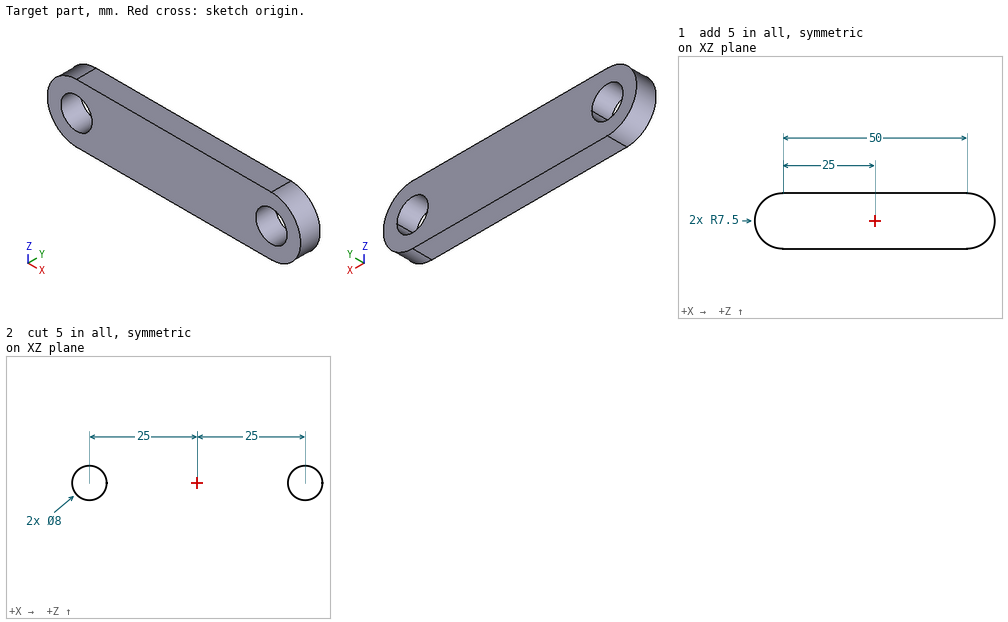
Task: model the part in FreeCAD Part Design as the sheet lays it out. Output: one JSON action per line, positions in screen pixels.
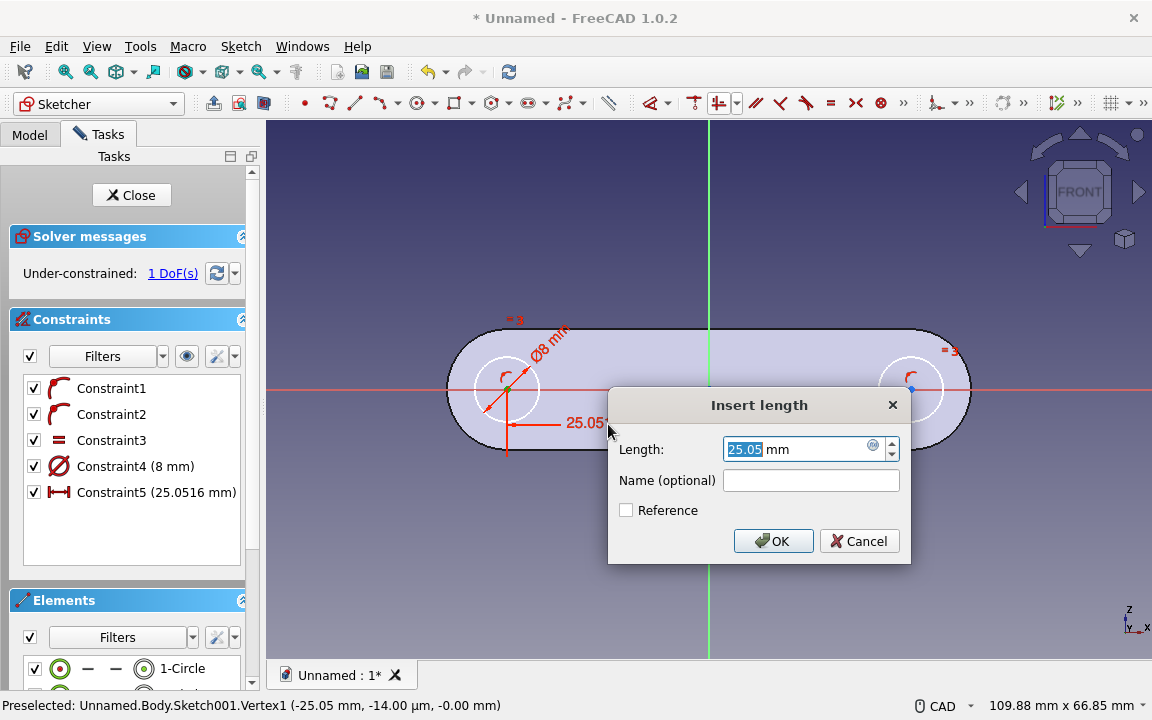
{"action": "type", "text": "25"}
{"action": "key", "text": "Return"}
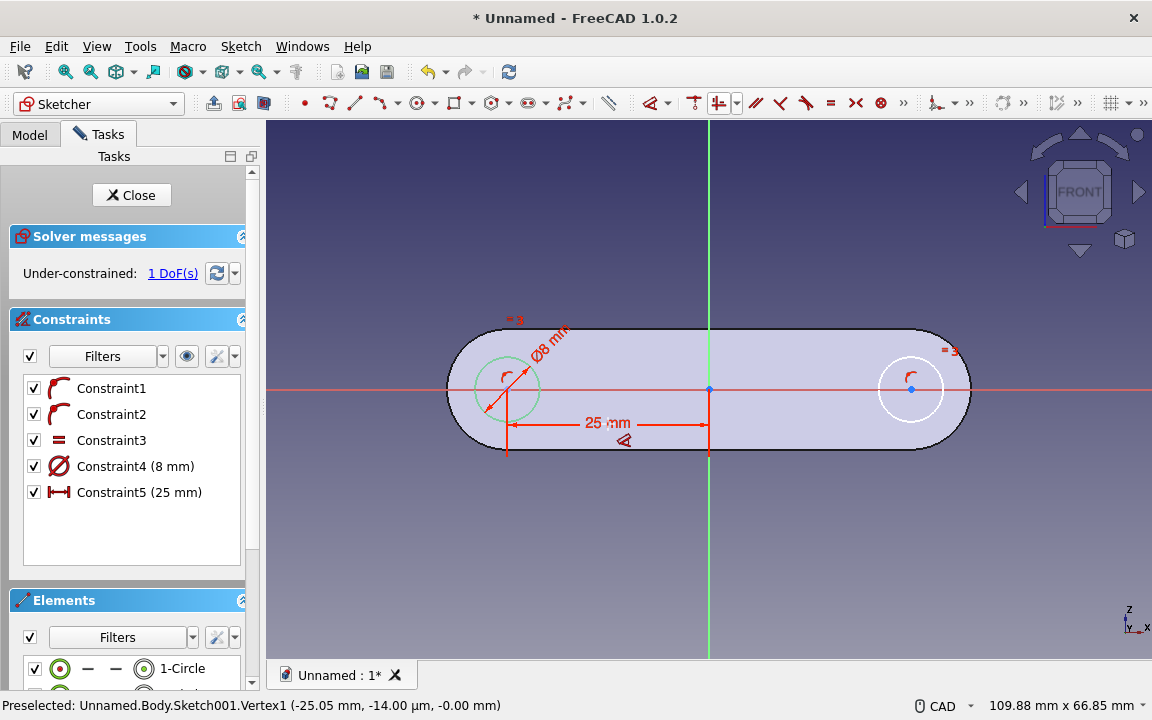
{"action": "left_click", "coordinate": [911, 390]}
{"action": "left_click", "coordinate": [810, 424]}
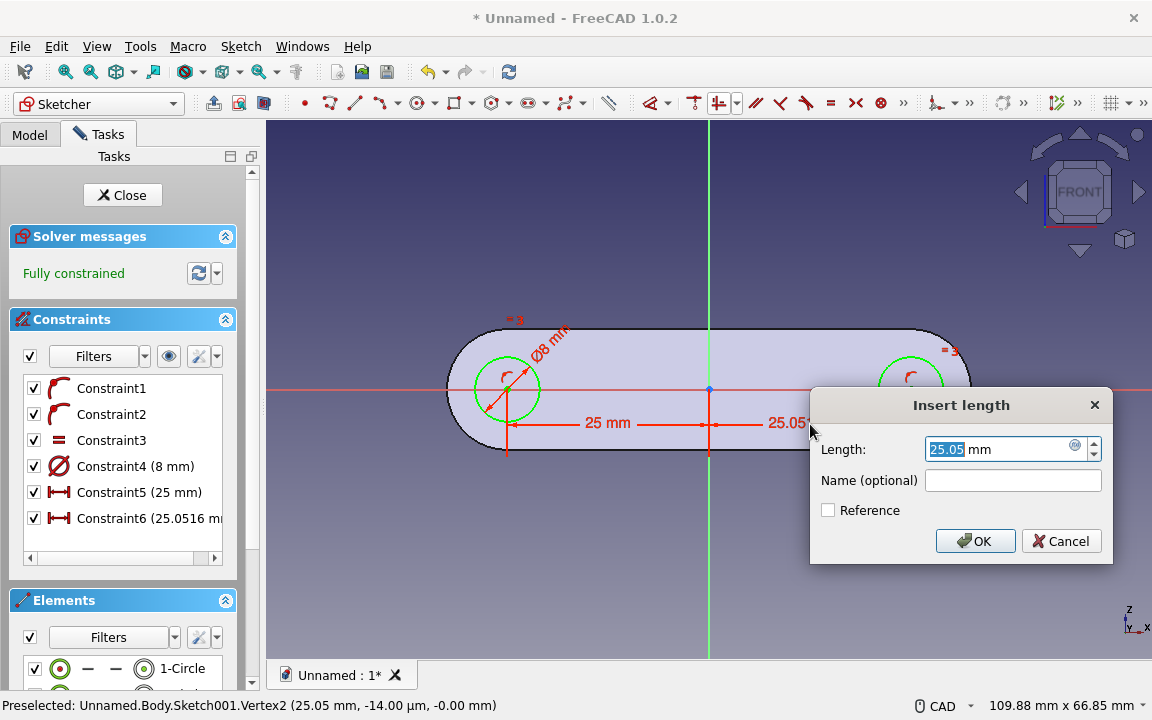
{"action": "type", "text": "25"}
{"action": "key", "text": "Return"}
{"action": "key", "text": "Escape"}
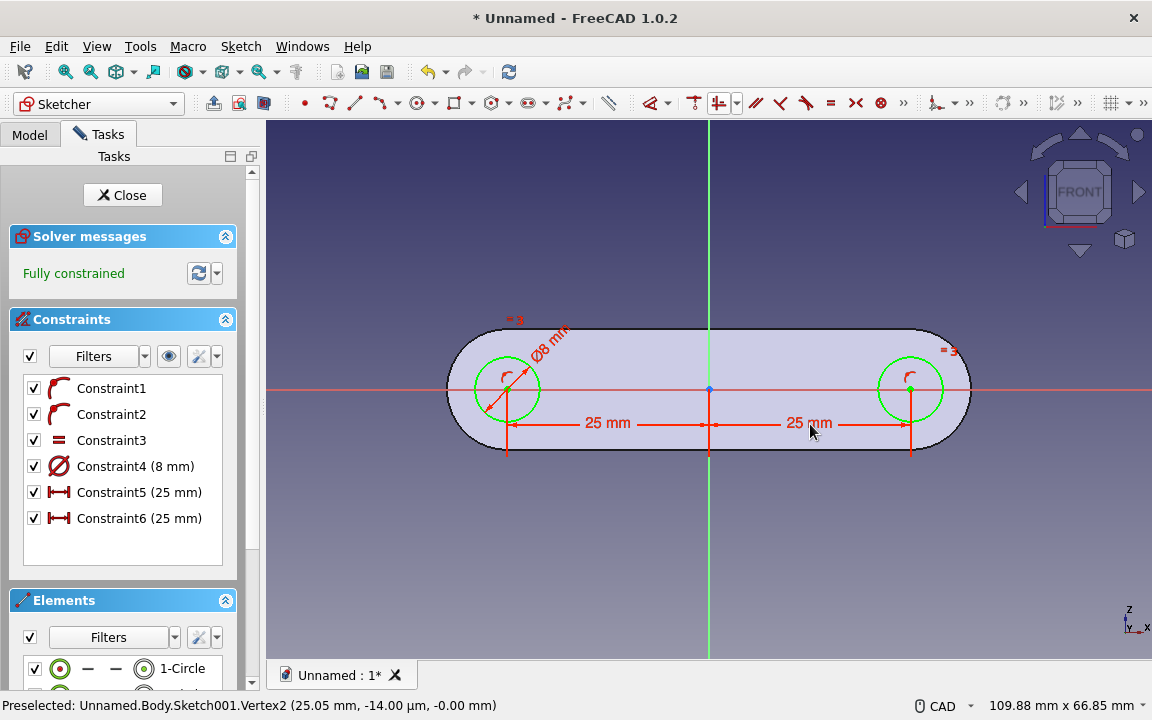
{"action": "left_click", "coordinate": [123, 195]}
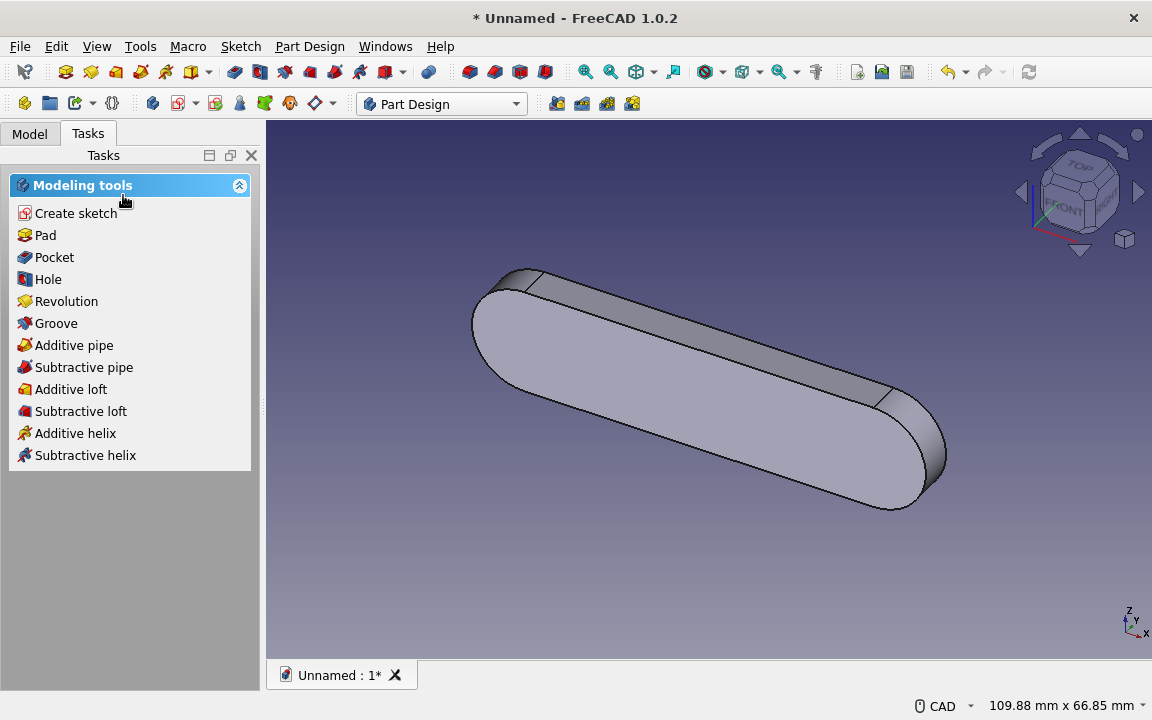
{"action": "left_click", "coordinate": [235, 72]}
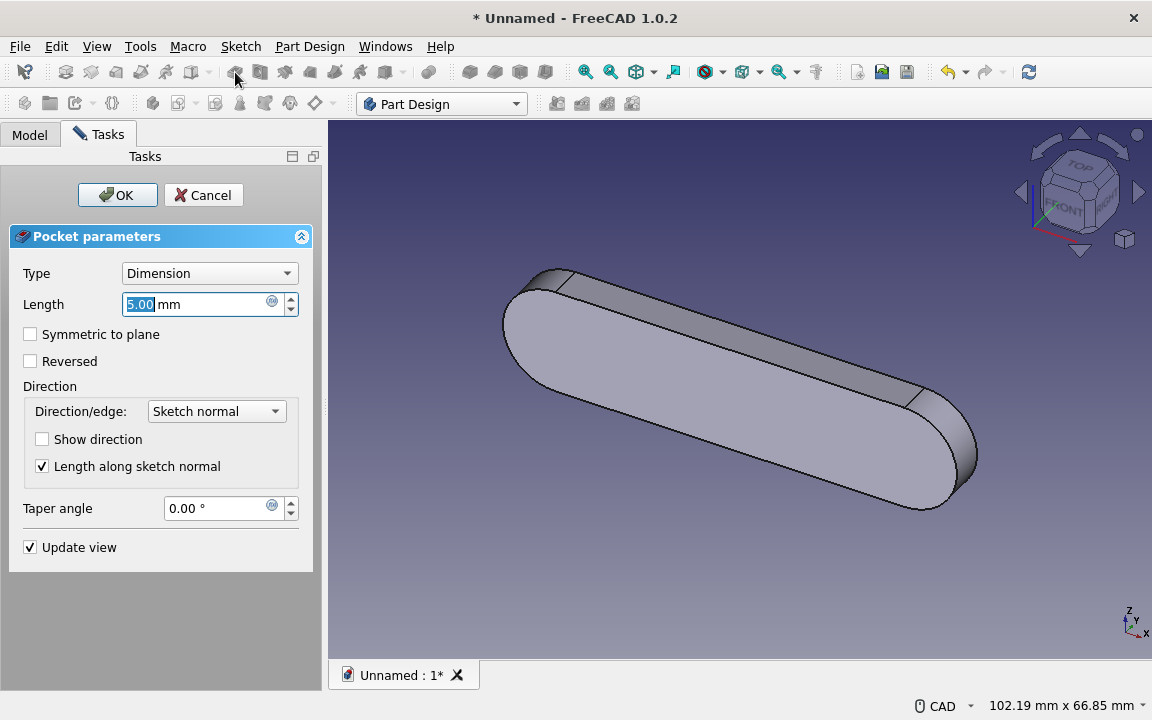
{"action": "type", "text": "5"}
{"action": "key", "text": "Tab"}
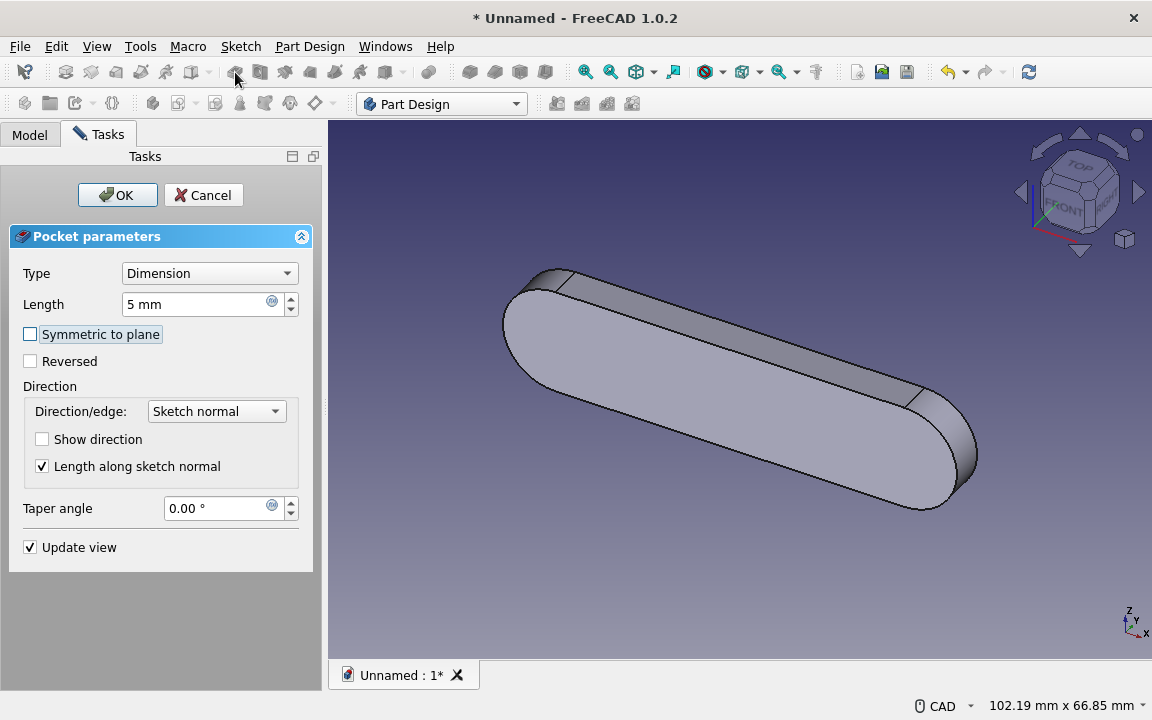
{"action": "left_click", "coordinate": [31, 334]}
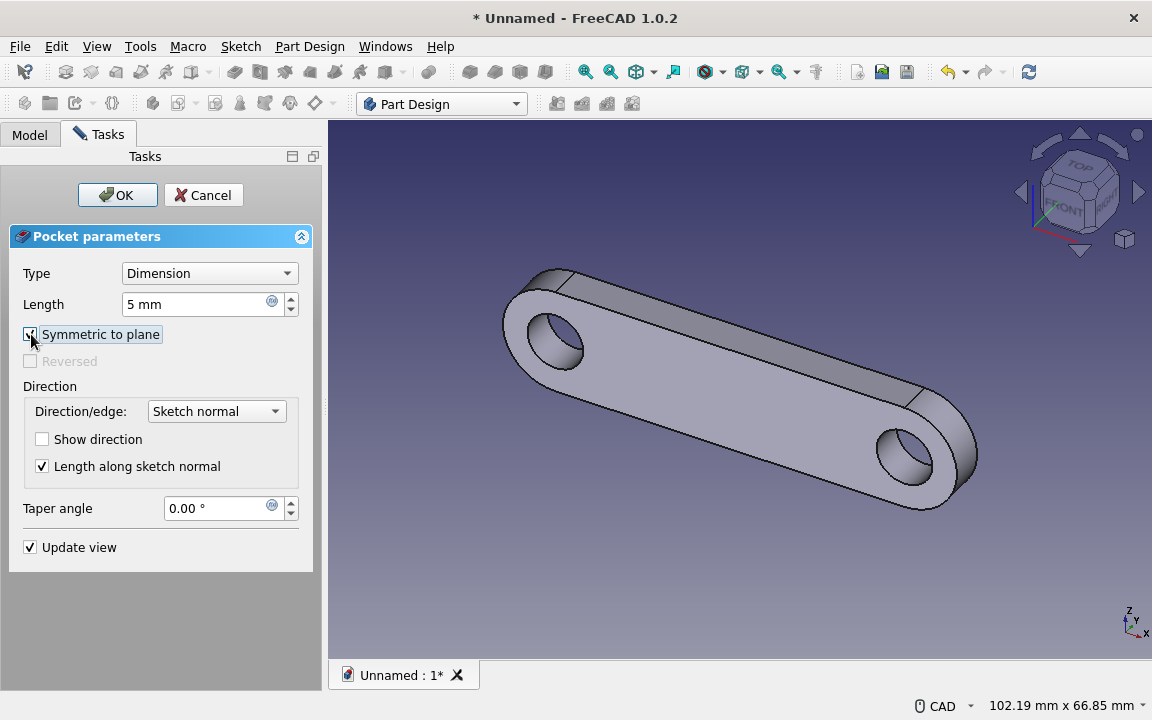
{"action": "left_click", "coordinate": [118, 195]}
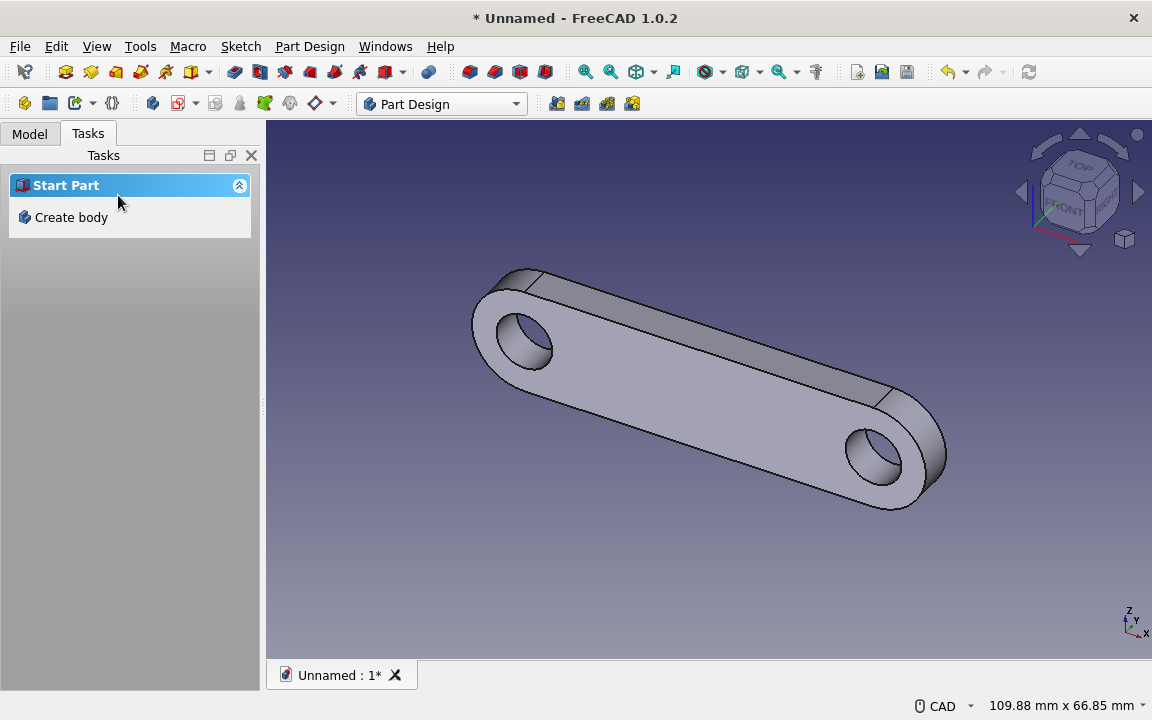
{"action": "key", "text": "0"}